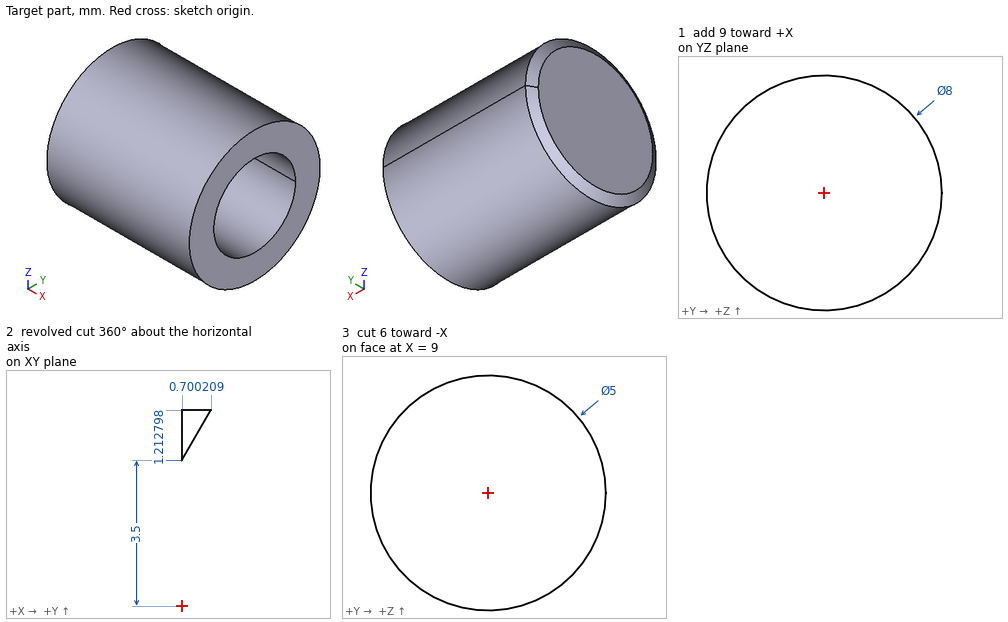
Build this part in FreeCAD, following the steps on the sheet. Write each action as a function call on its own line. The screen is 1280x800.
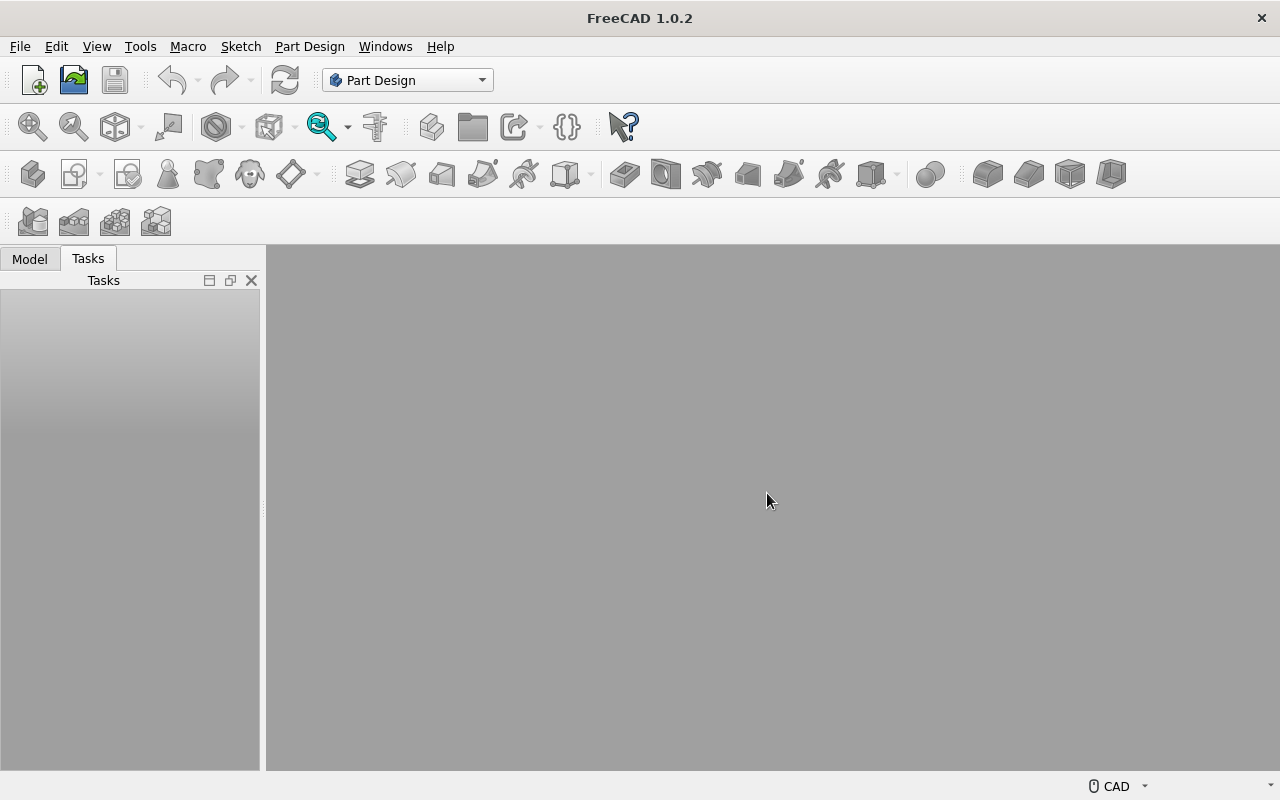
click(33, 80)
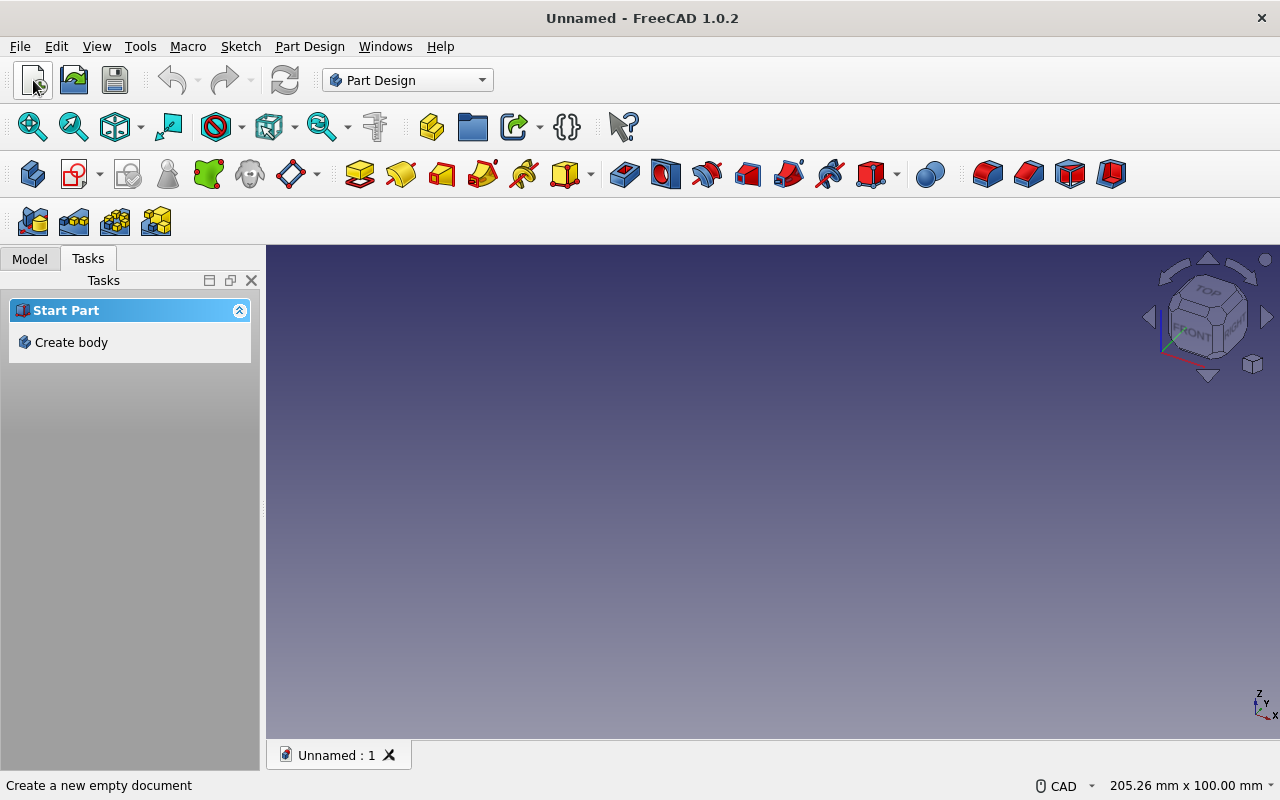
click(74, 174)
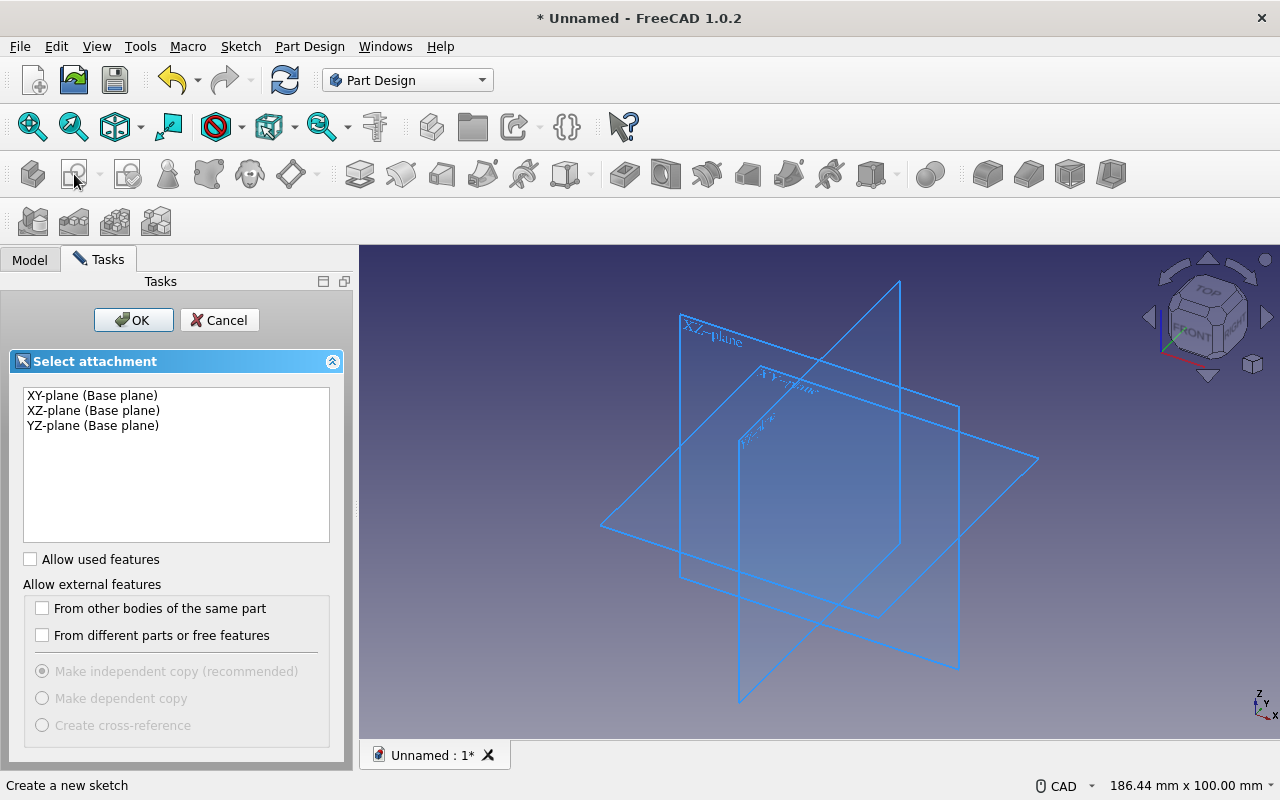
click(84, 426)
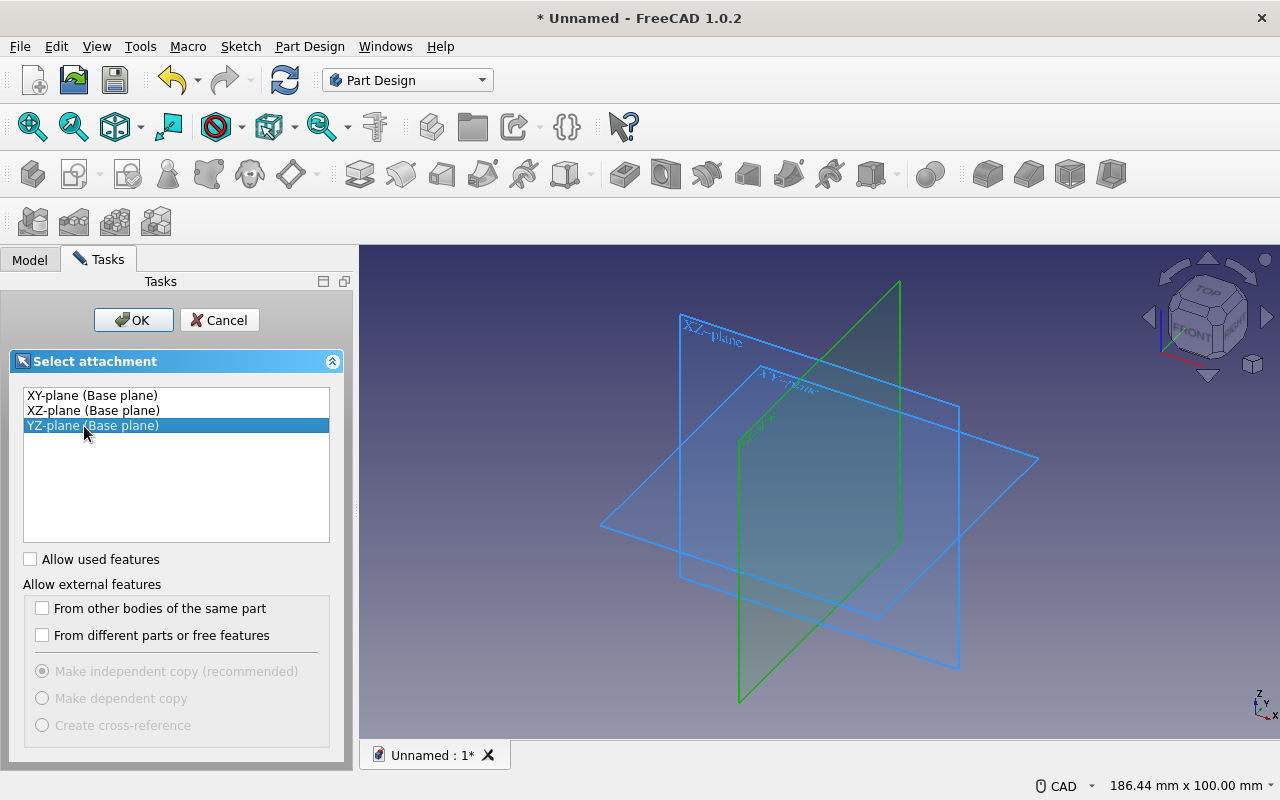
click(134, 320)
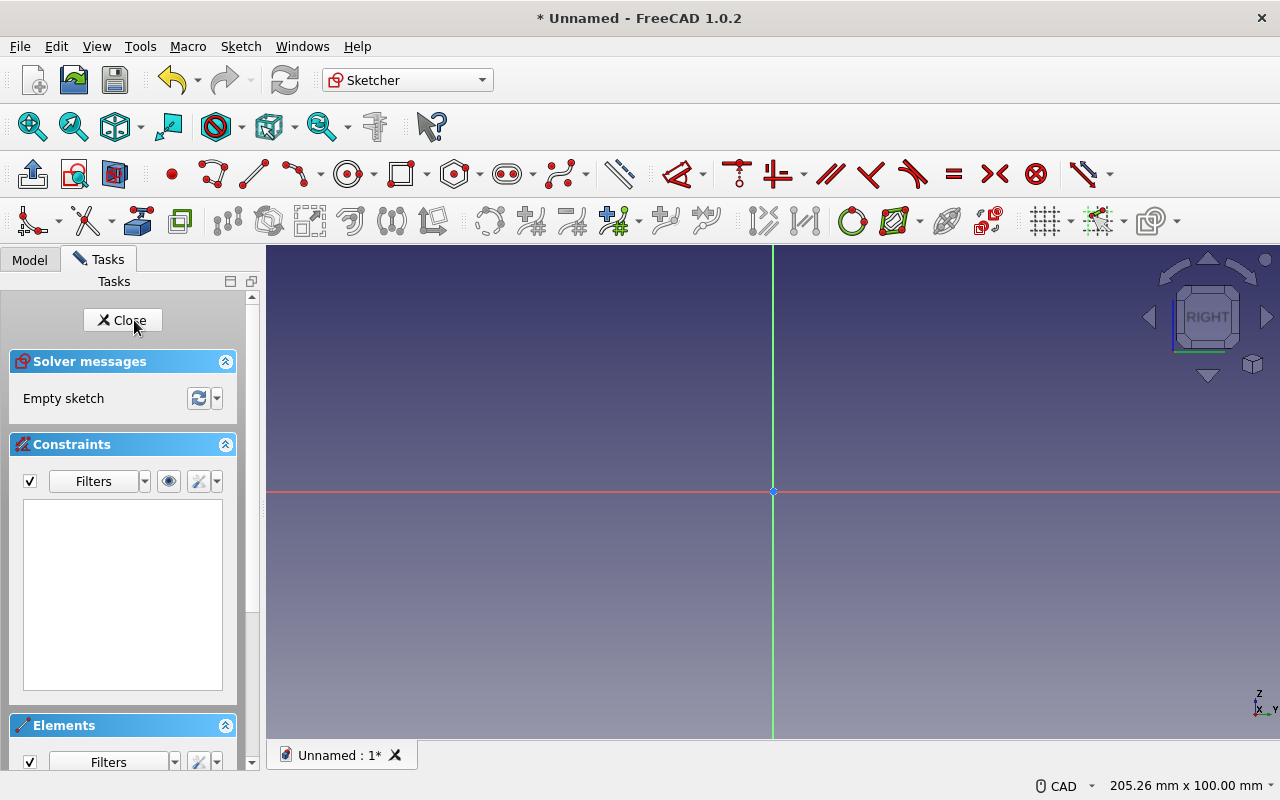
scroll(784, 492, up, 10)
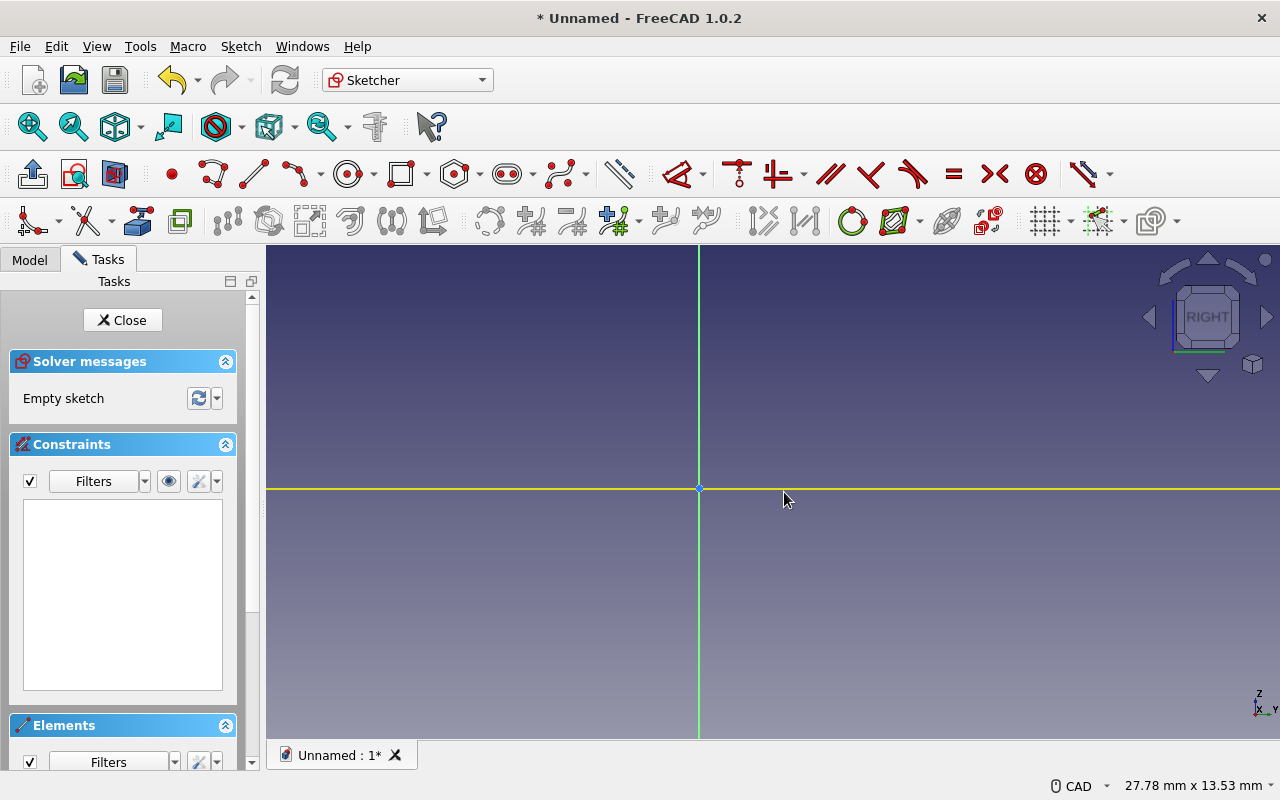
click(348, 174)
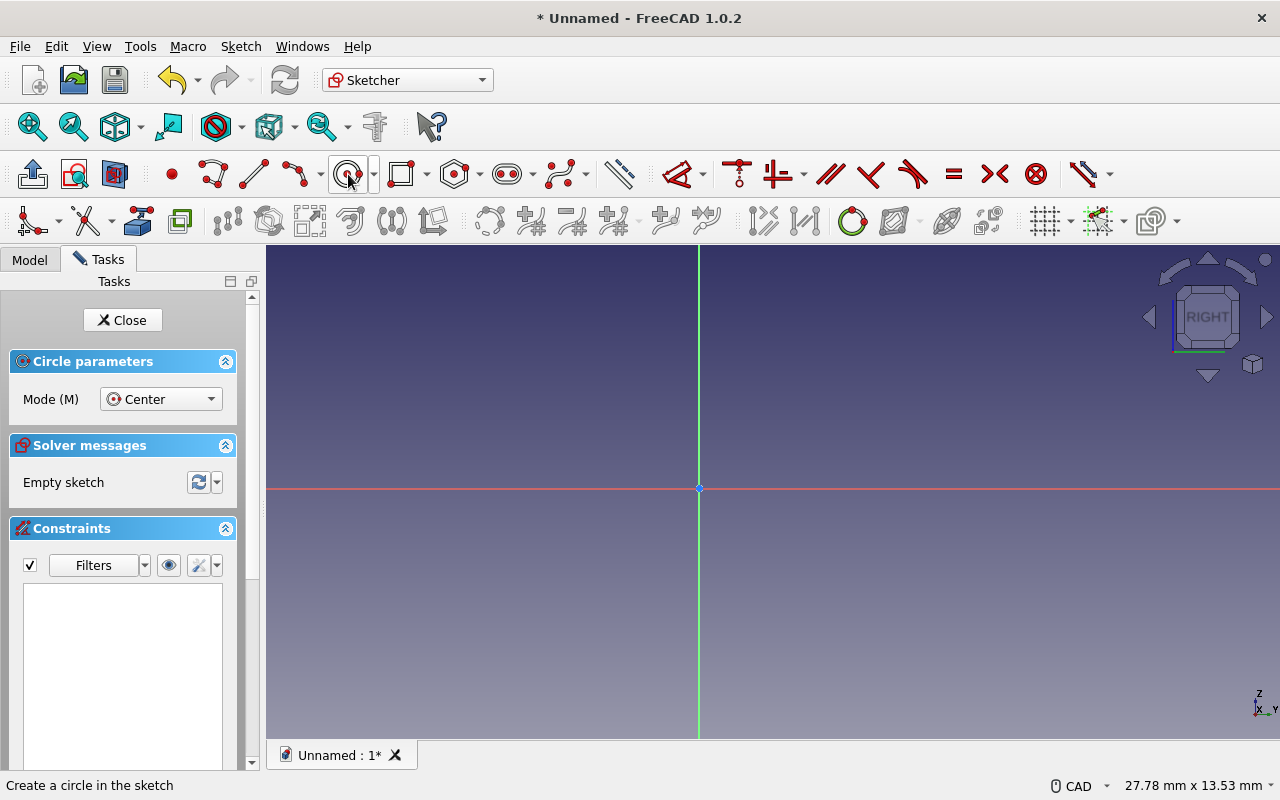
click(699, 489)
click(803, 386)
key(Escape)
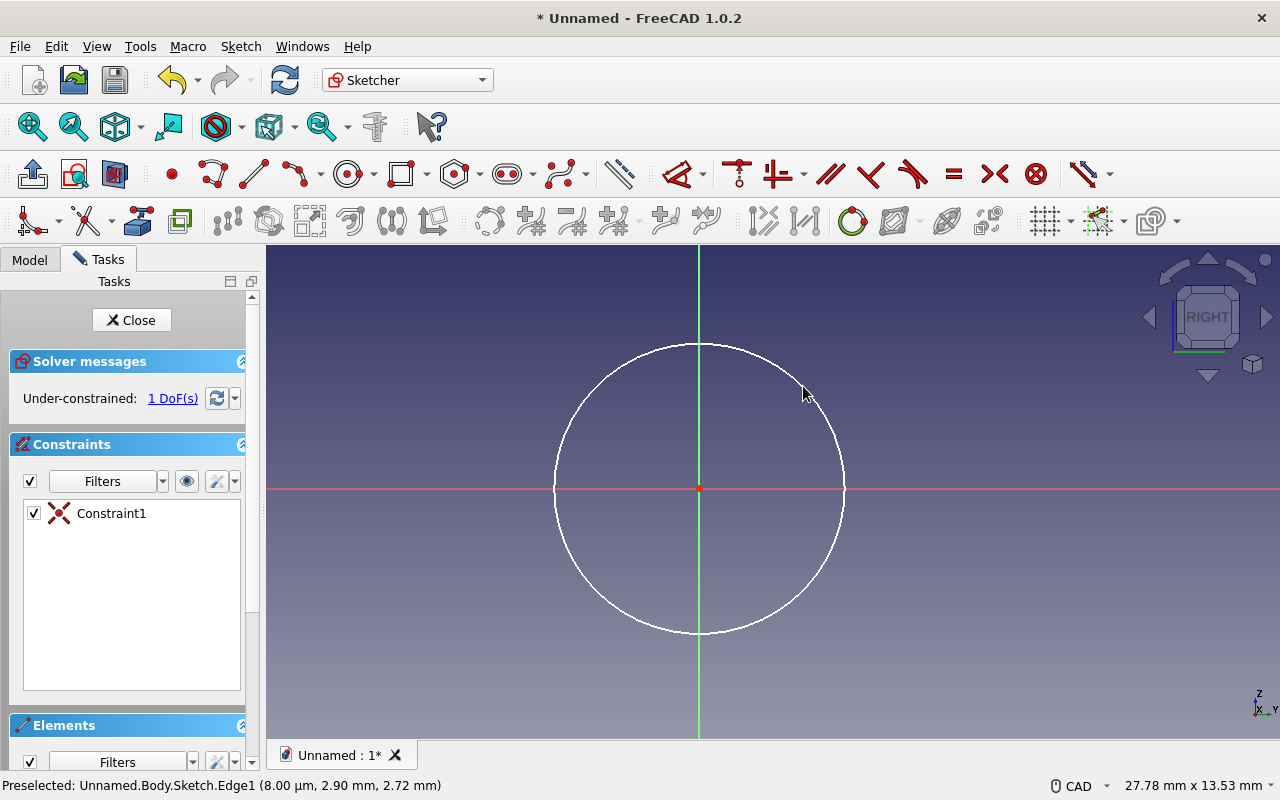
click(676, 174)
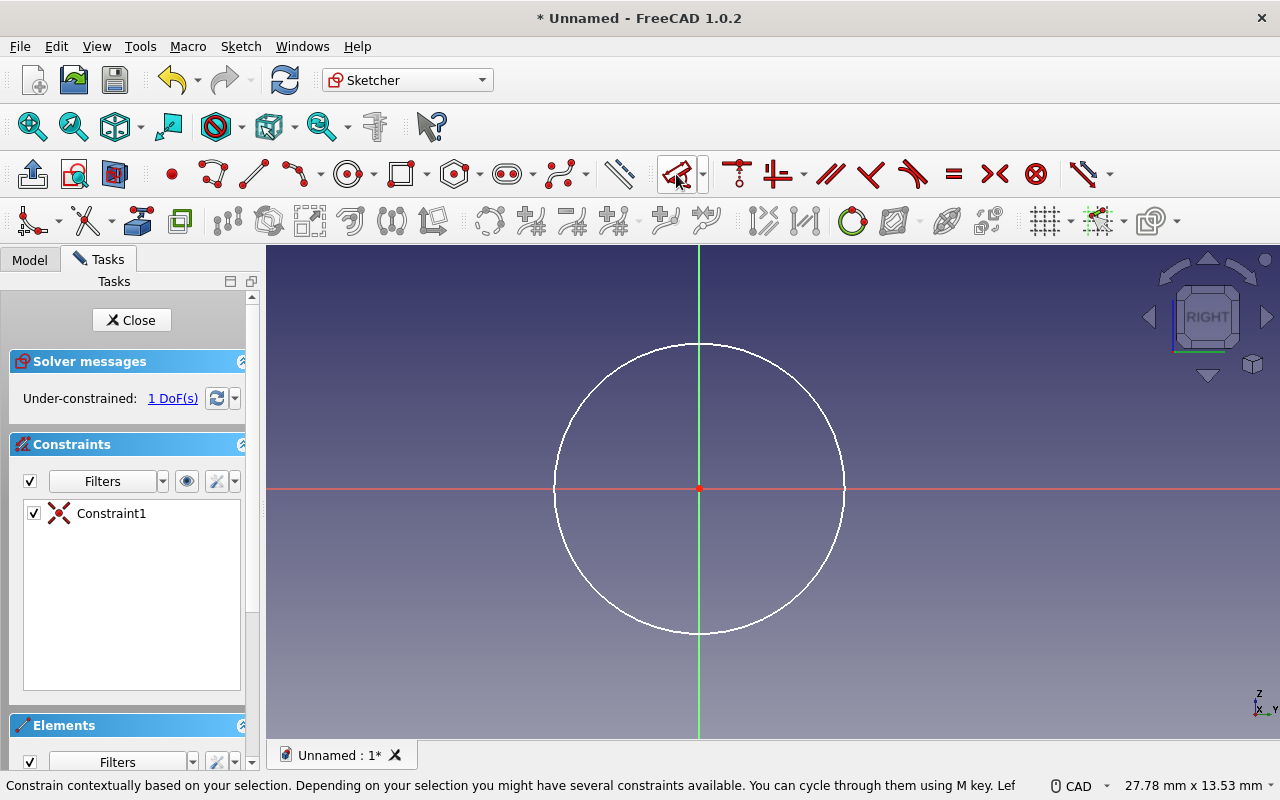
click(802, 386)
click(825, 363)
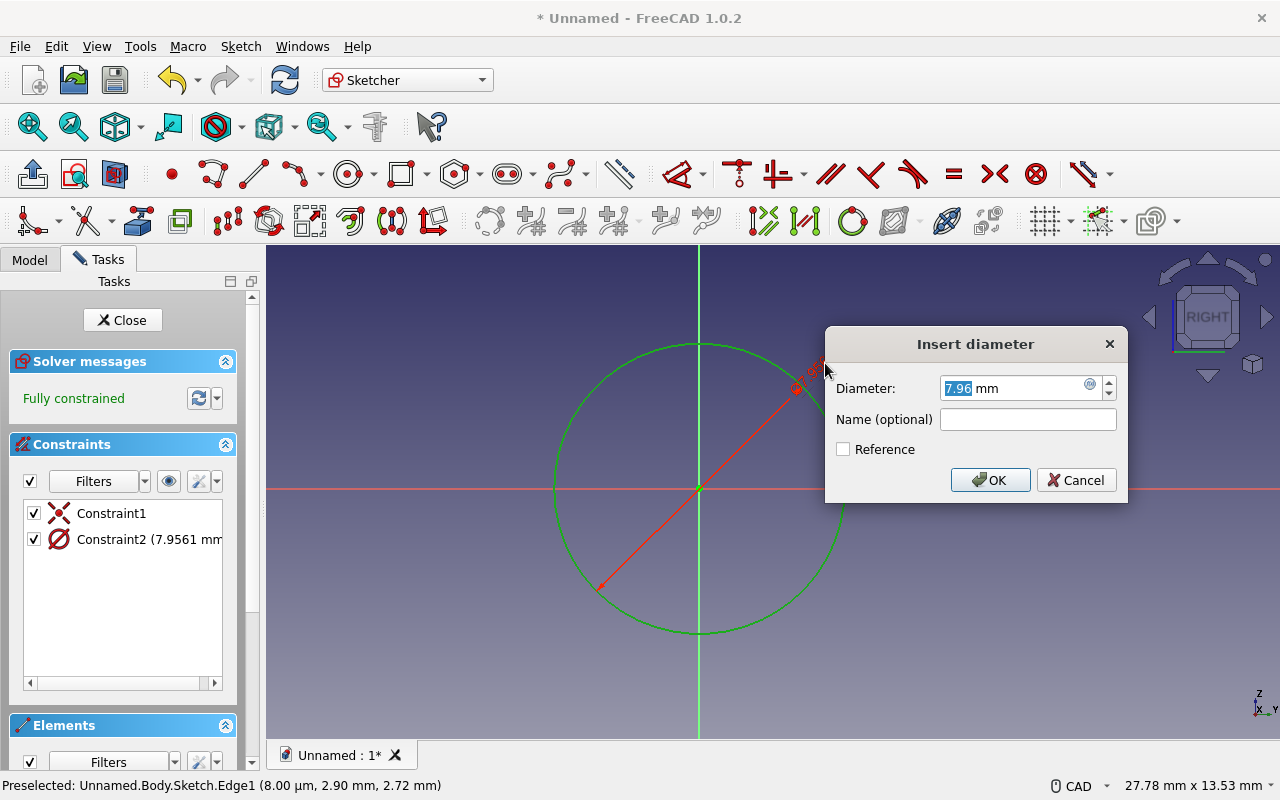
text(8)
key(Return)
key(Escape)